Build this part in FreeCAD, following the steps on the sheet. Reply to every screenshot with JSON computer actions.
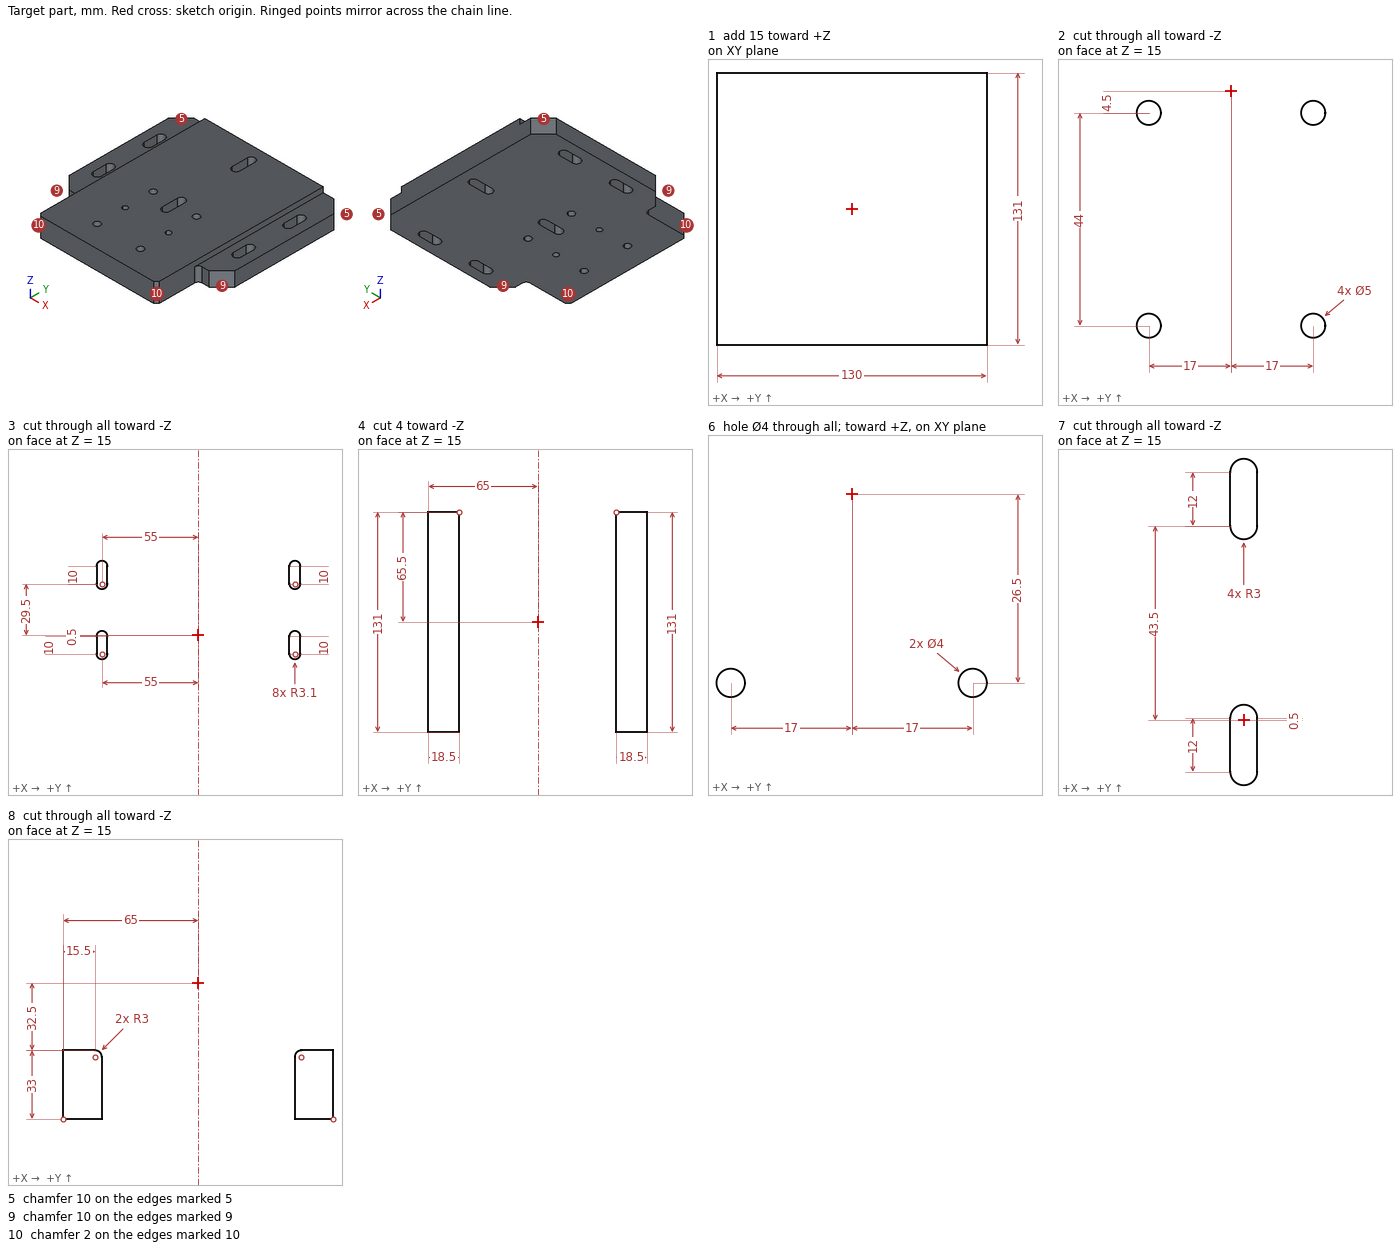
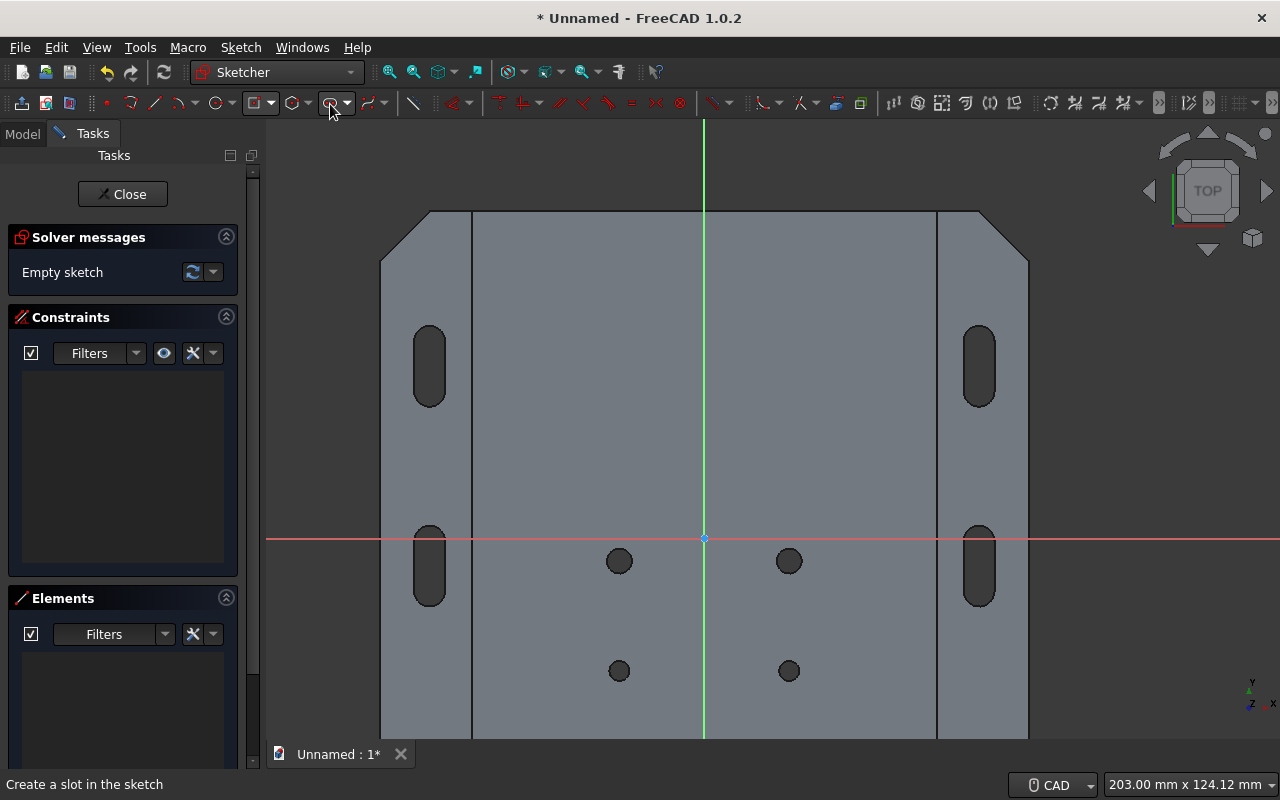
{"action": "scroll", "coordinate": [704, 321], "scroll_direction": "up", "scroll_amount": 3}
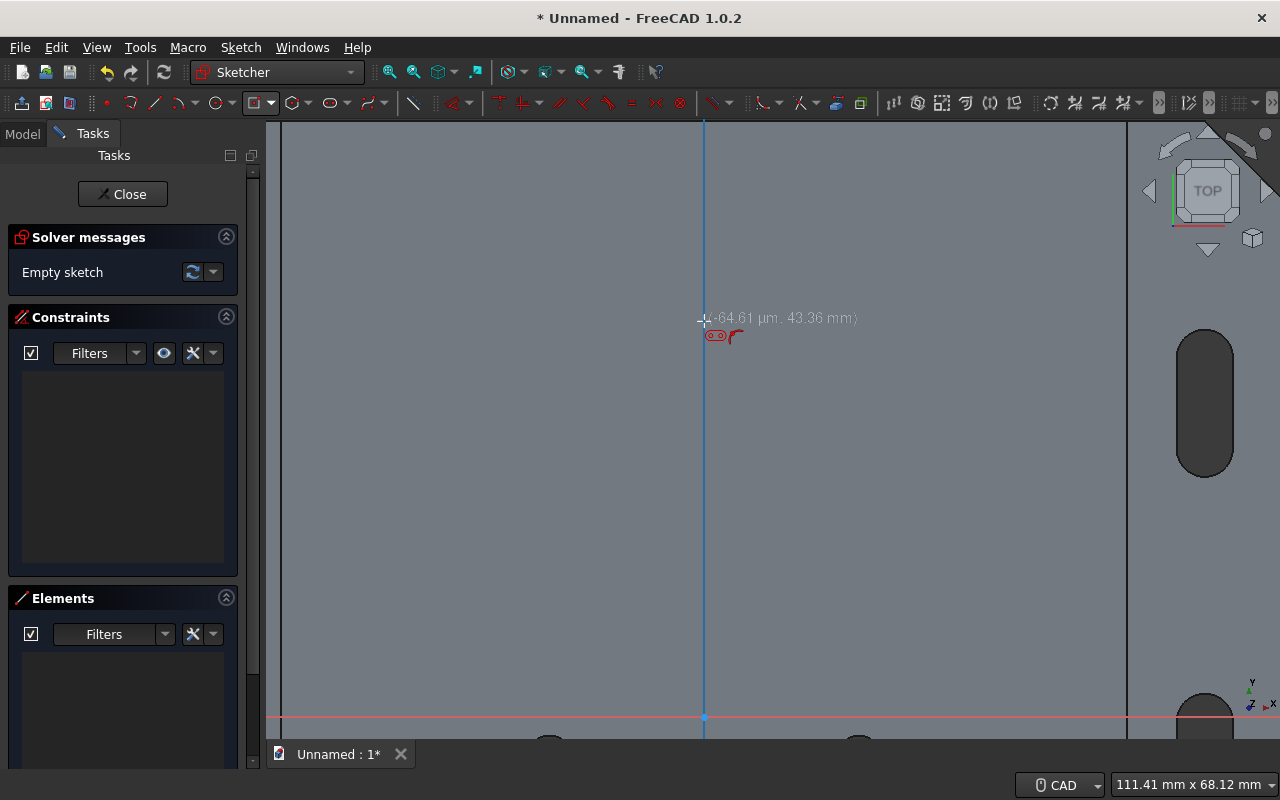
{"action": "left_click", "coordinate": [704, 321]}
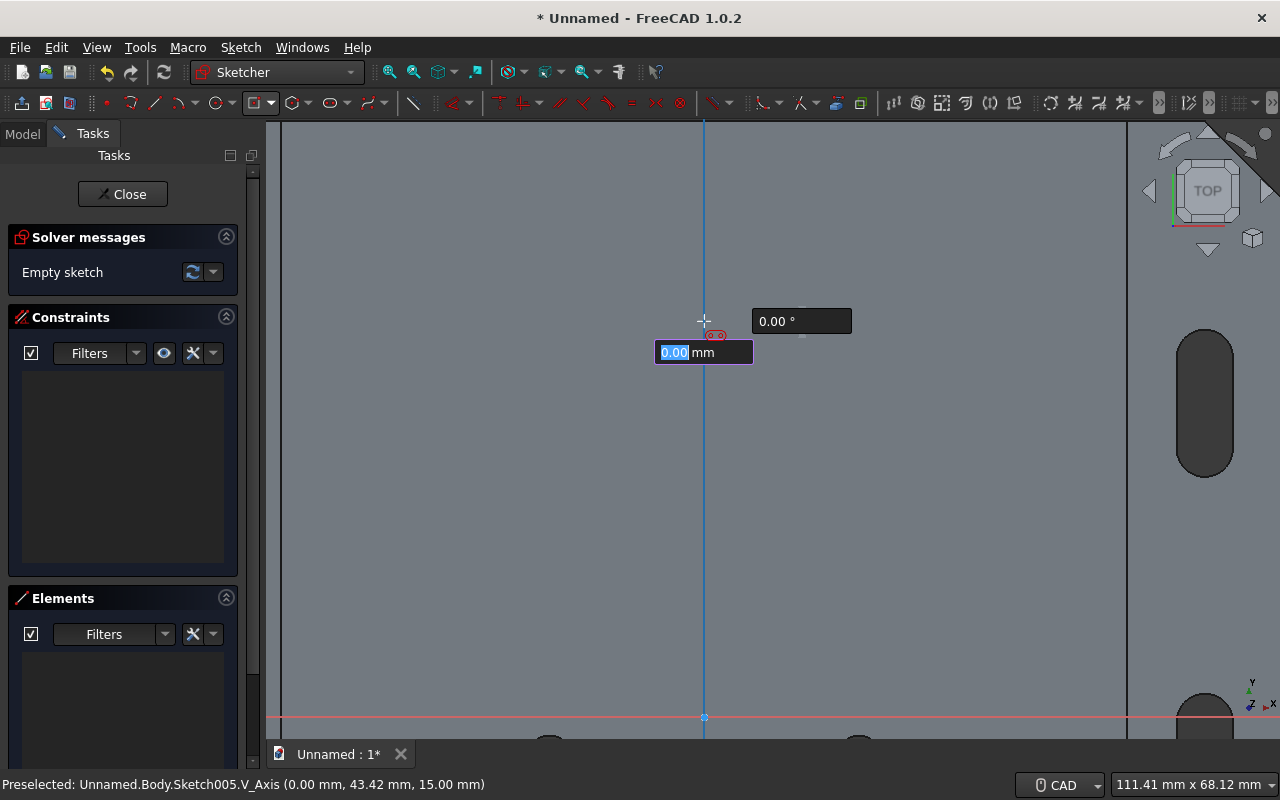
{"action": "left_click", "coordinate": [713, 212]}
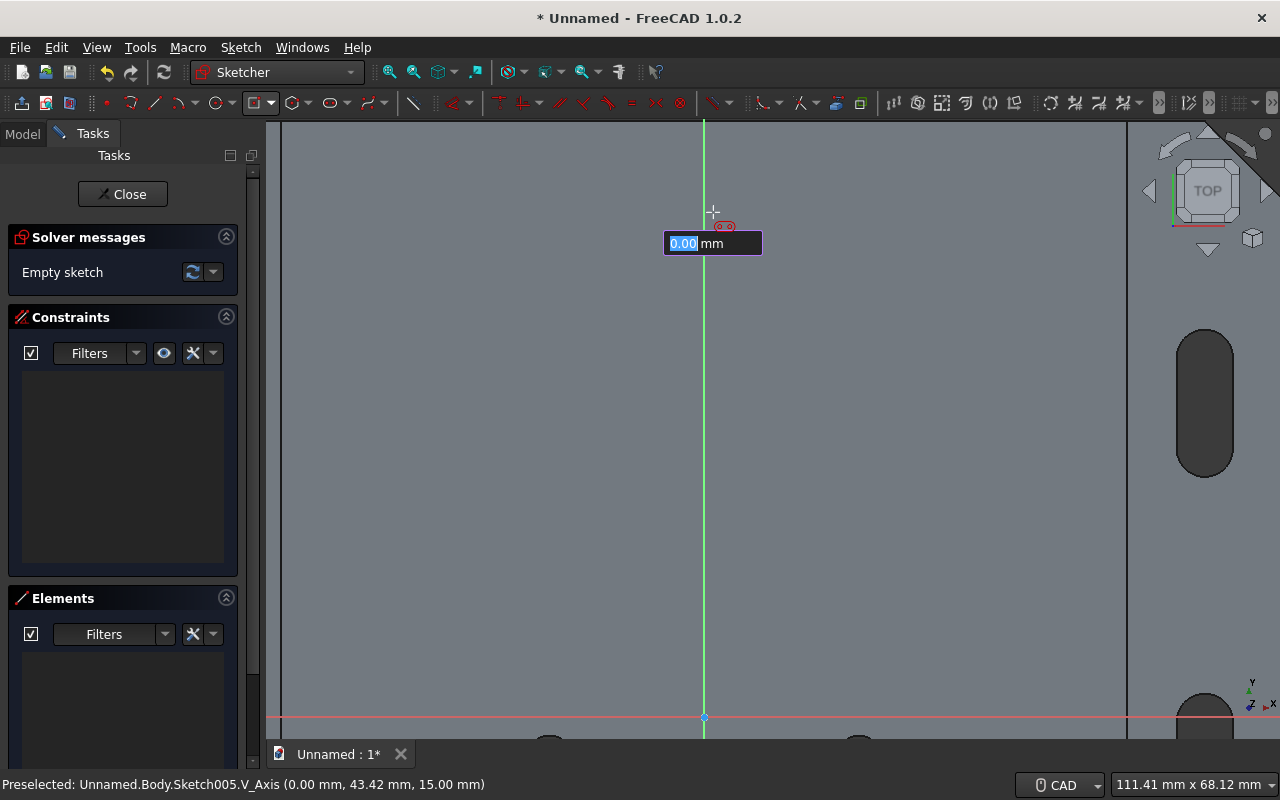
{"action": "left_click", "coordinate": [677, 267]}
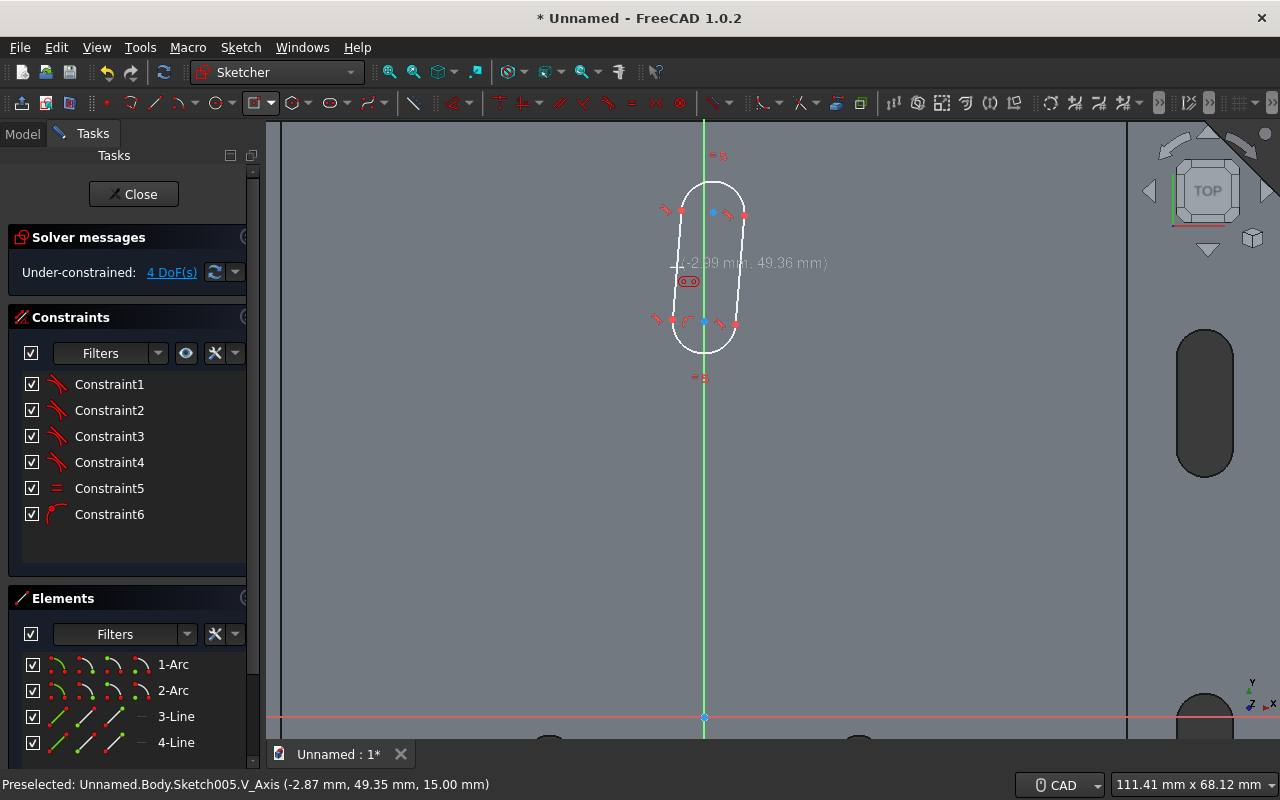
{"action": "scroll", "coordinate": [705, 322], "scroll_direction": "down", "scroll_amount": 3}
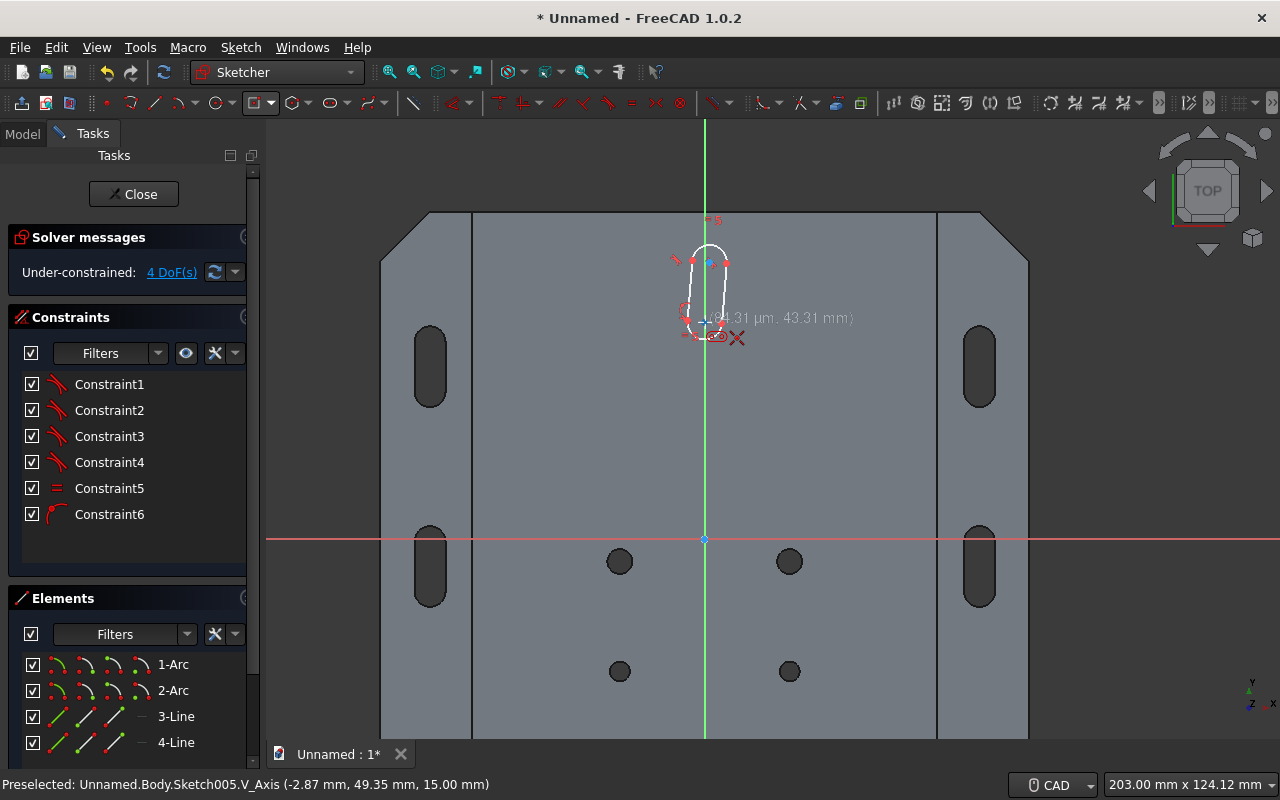
{"action": "scroll", "coordinate": [705, 597], "scroll_direction": "up", "scroll_amount": 3}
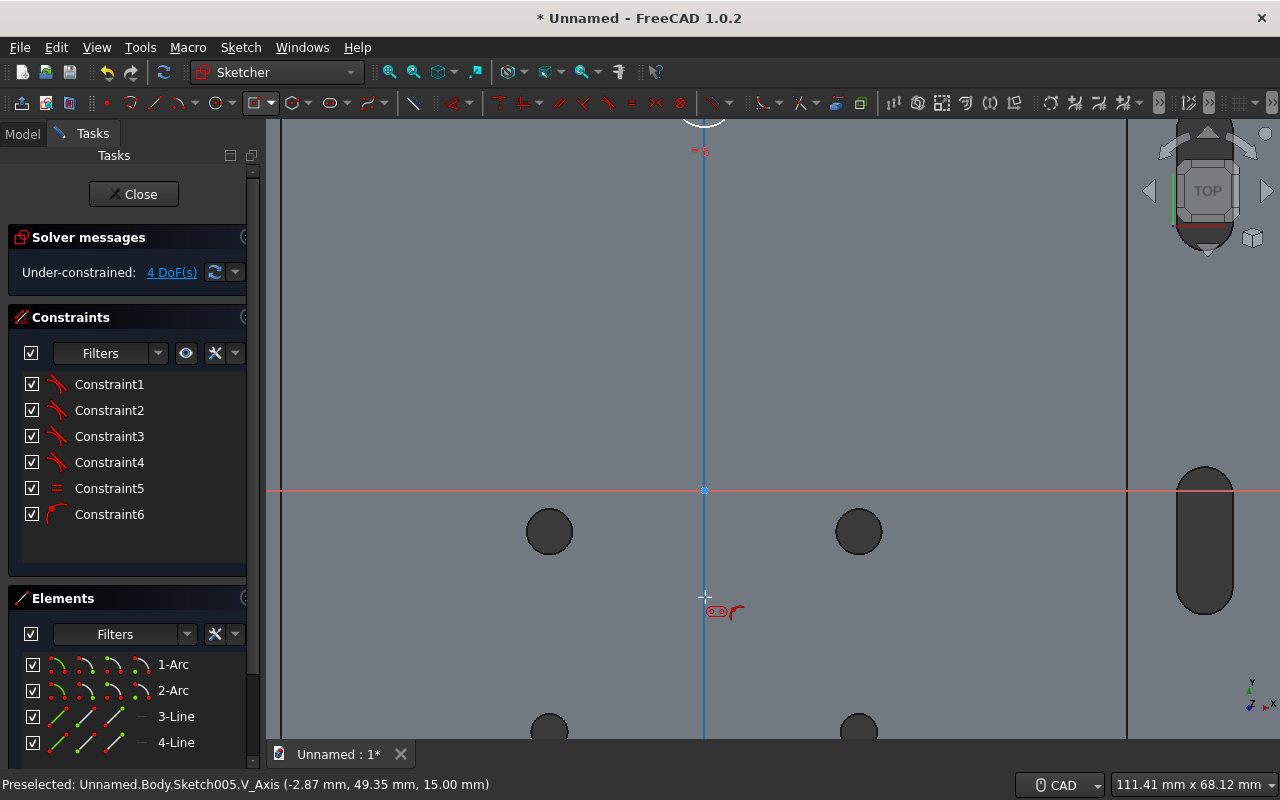
{"action": "left_click", "coordinate": [704, 595]}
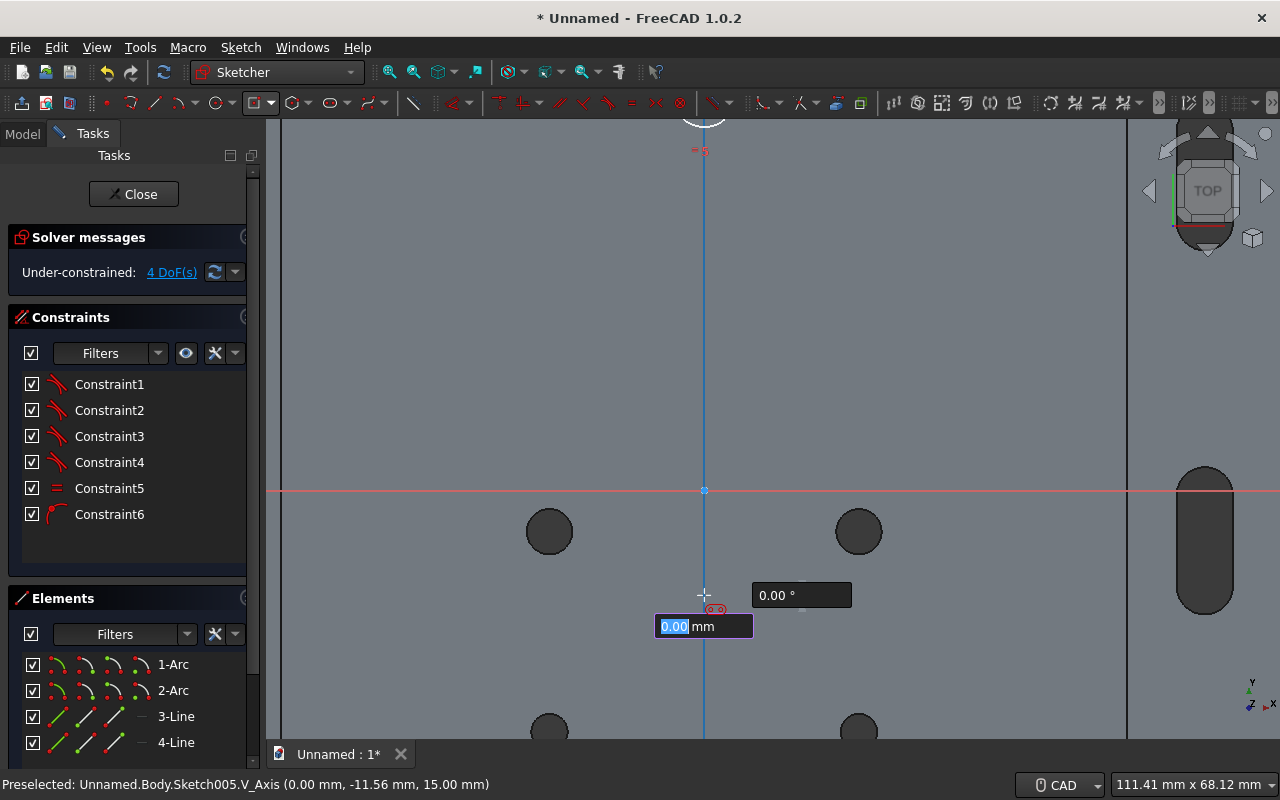
{"action": "scroll", "coordinate": [704, 486], "scroll_direction": "up", "scroll_amount": 7}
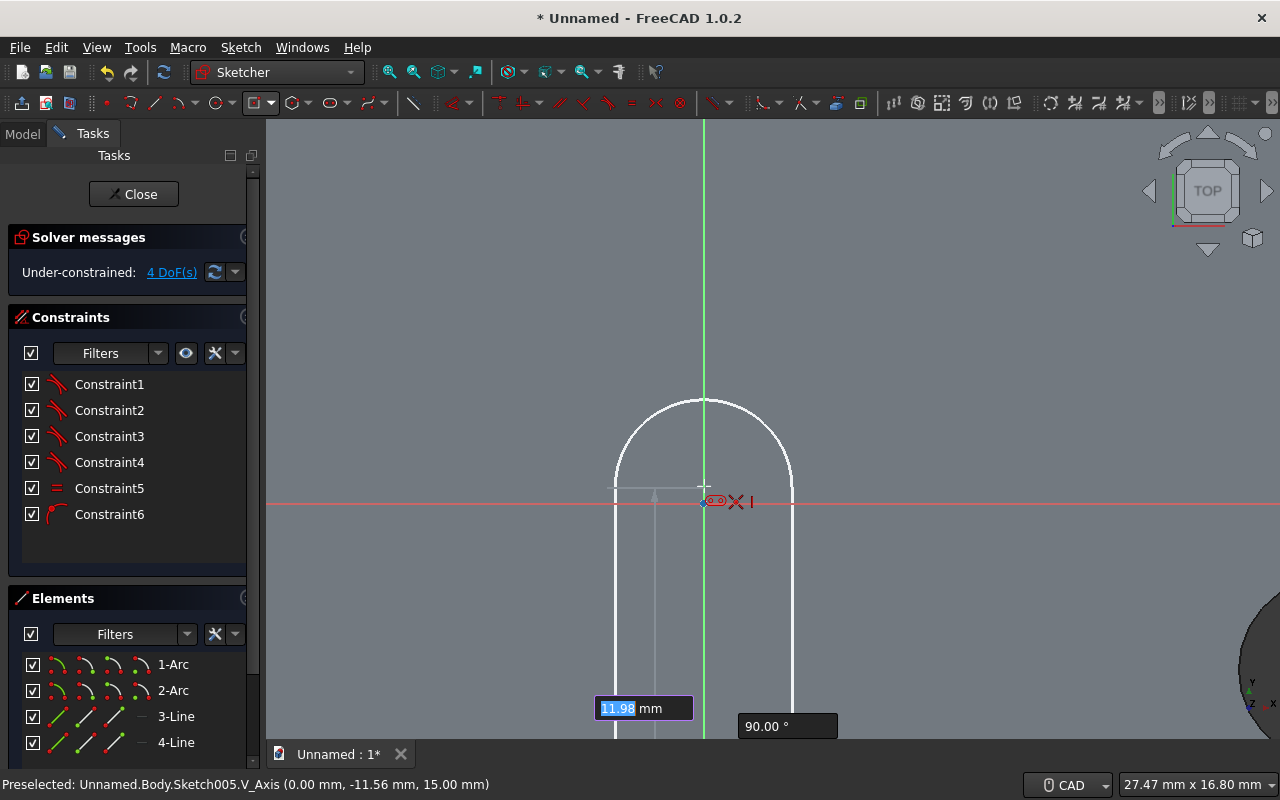
{"action": "left_click", "coordinate": [713, 485]}